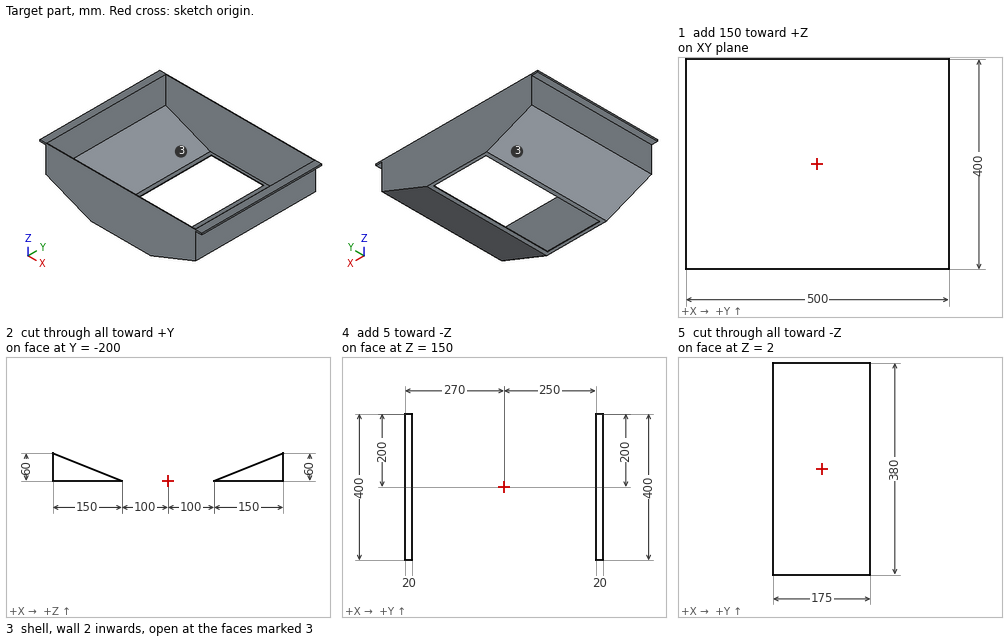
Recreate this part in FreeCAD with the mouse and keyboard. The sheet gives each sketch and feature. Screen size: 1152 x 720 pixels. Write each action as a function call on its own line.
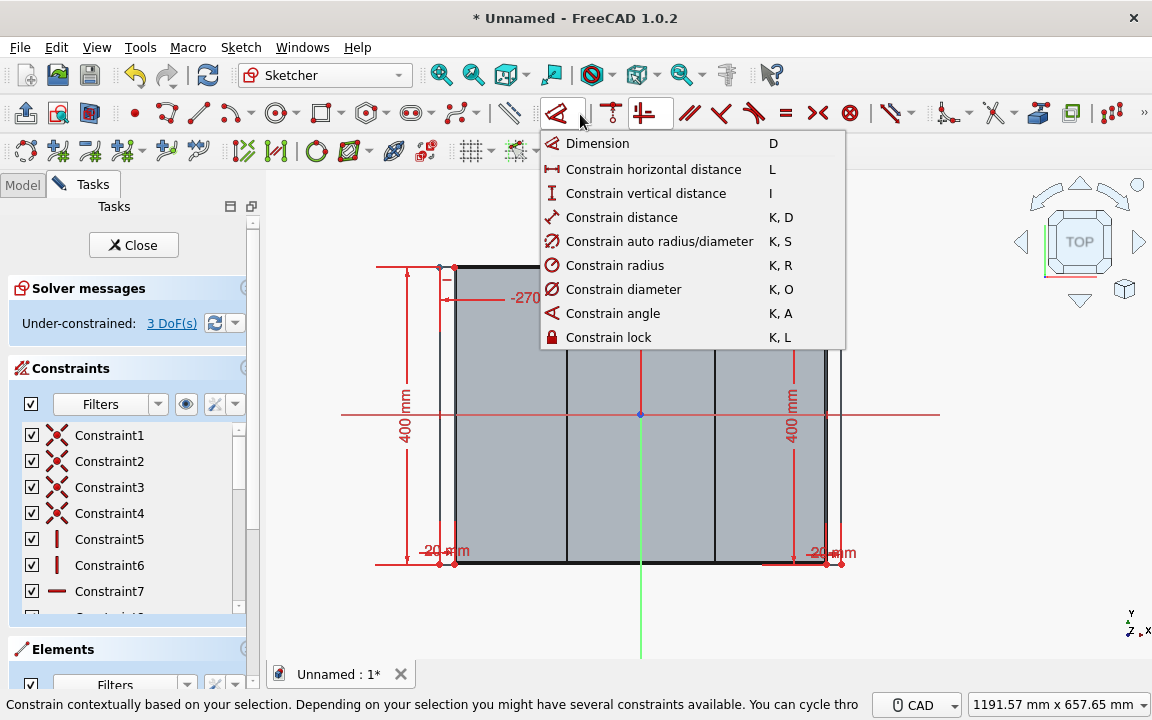
click(693, 193)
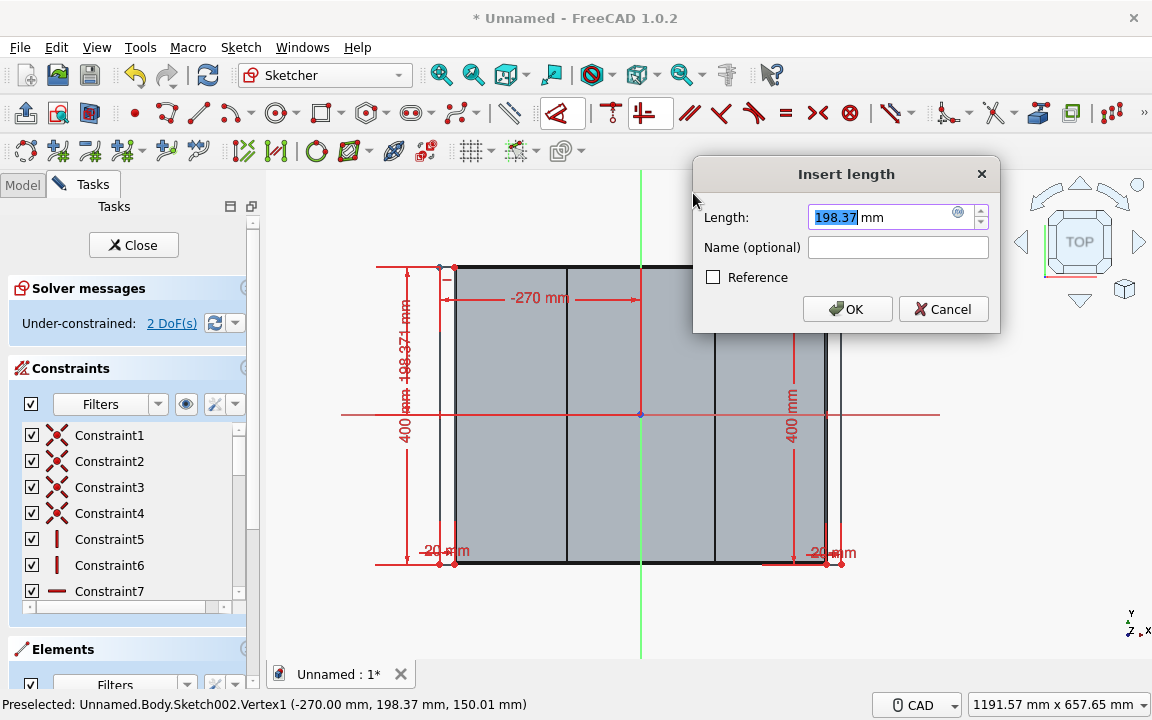
text(200)
key(Return)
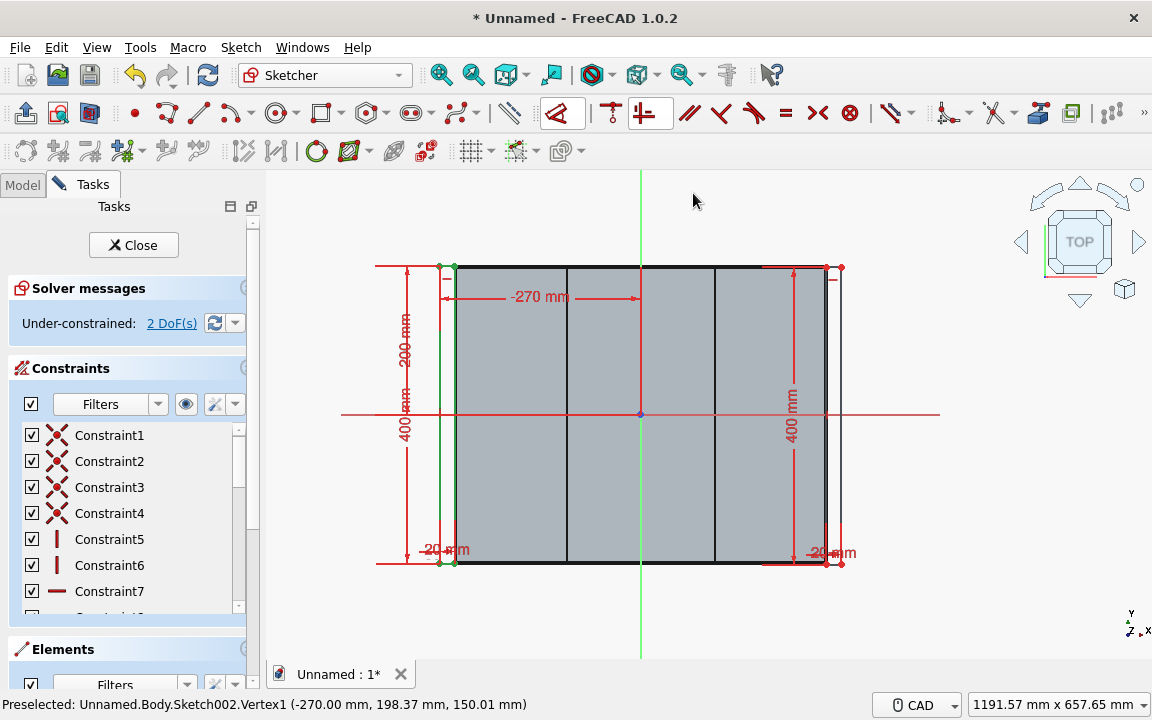
click(826, 267)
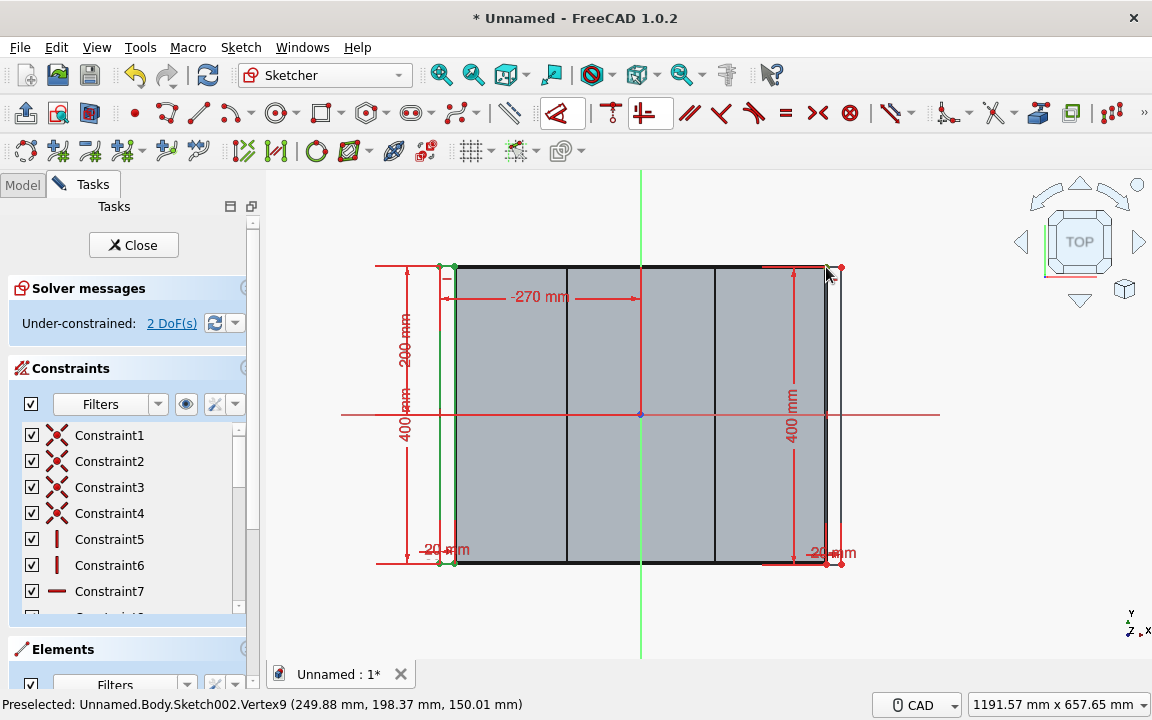
key(l)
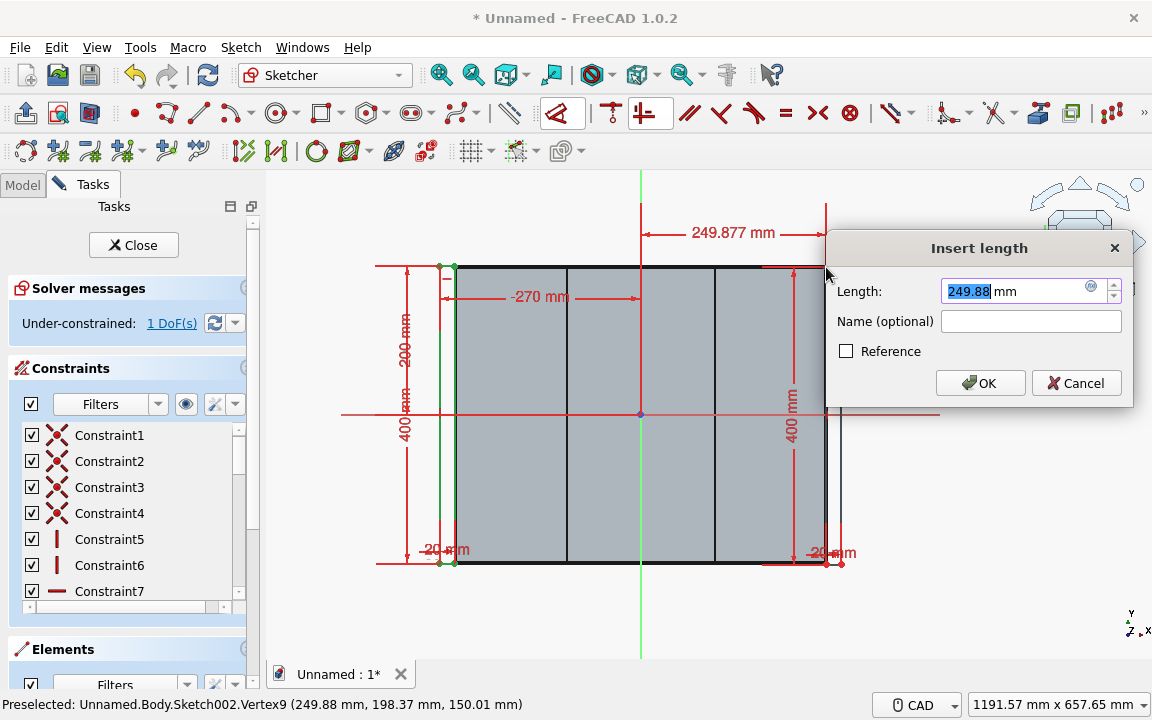
text(250)
key(Return)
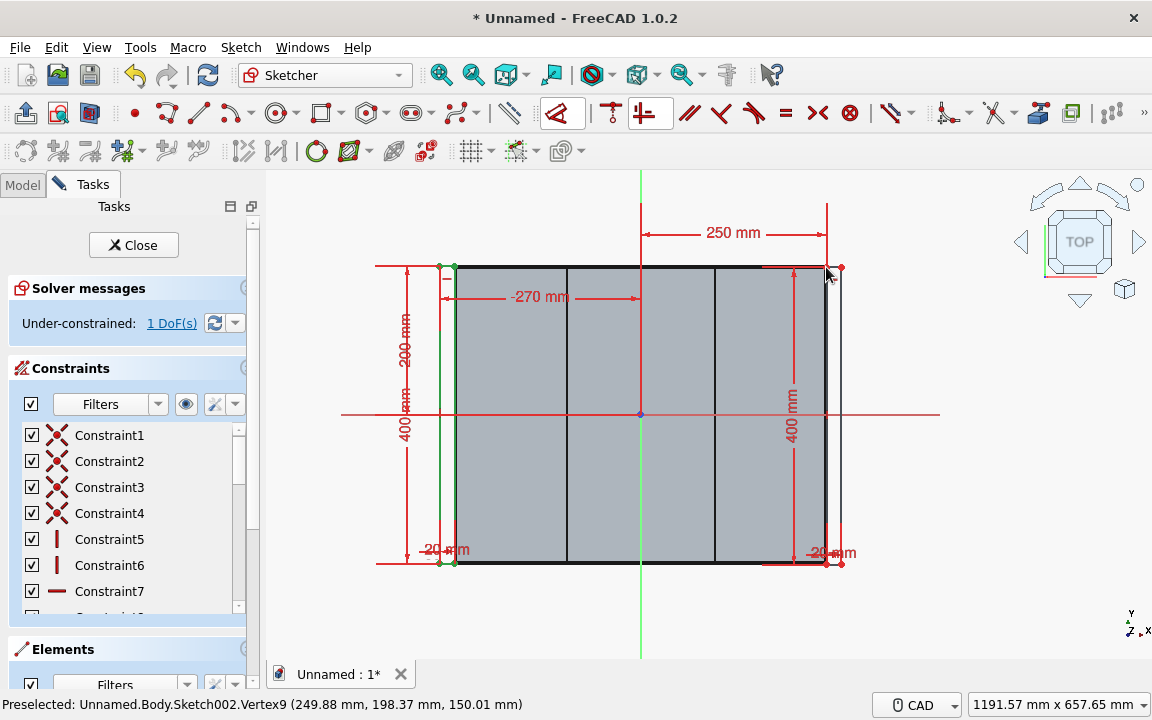
click(827, 267)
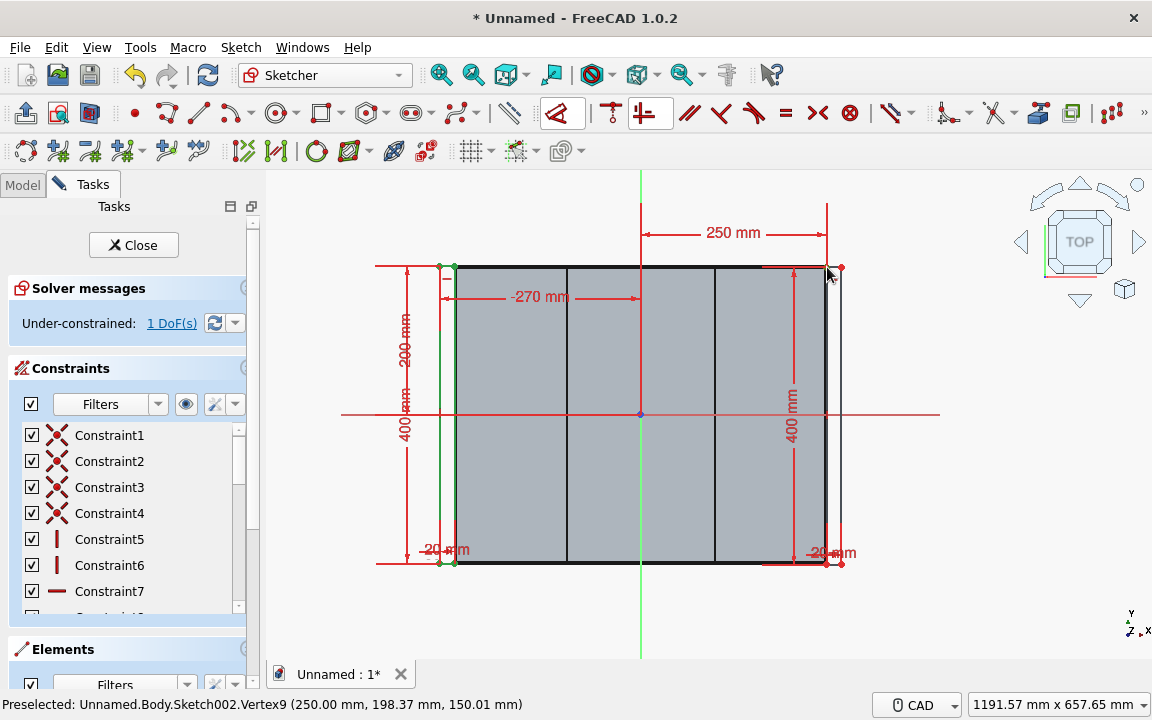
key(i)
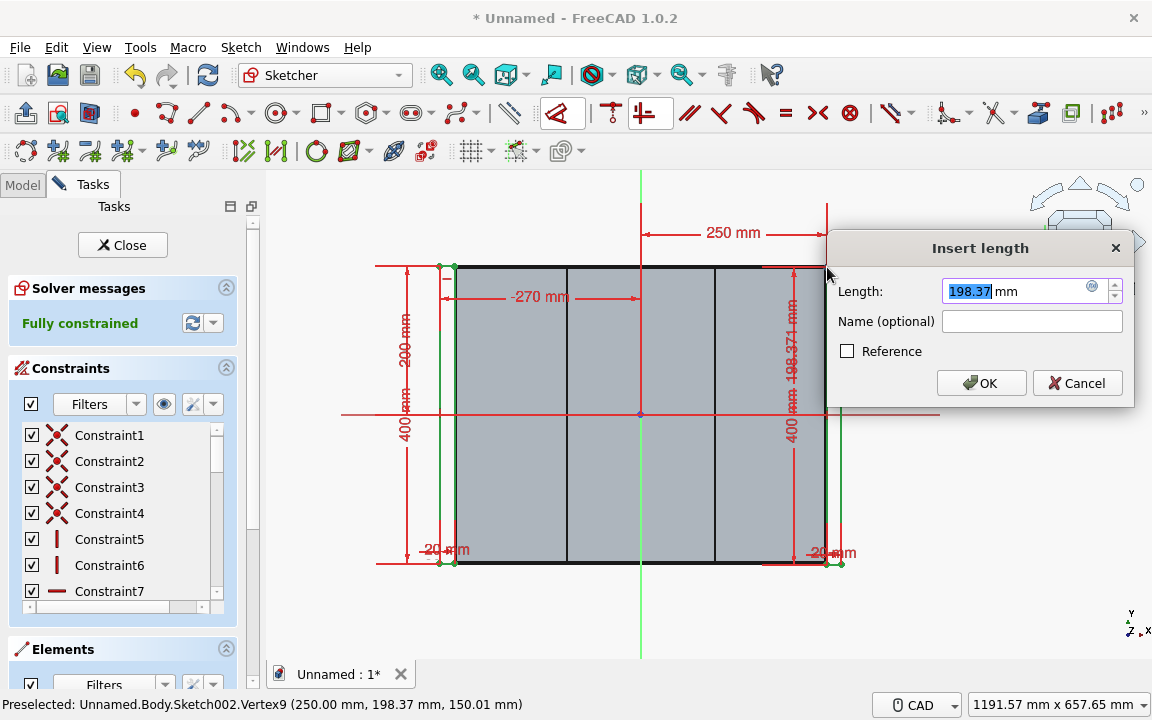
text(200)
key(Return)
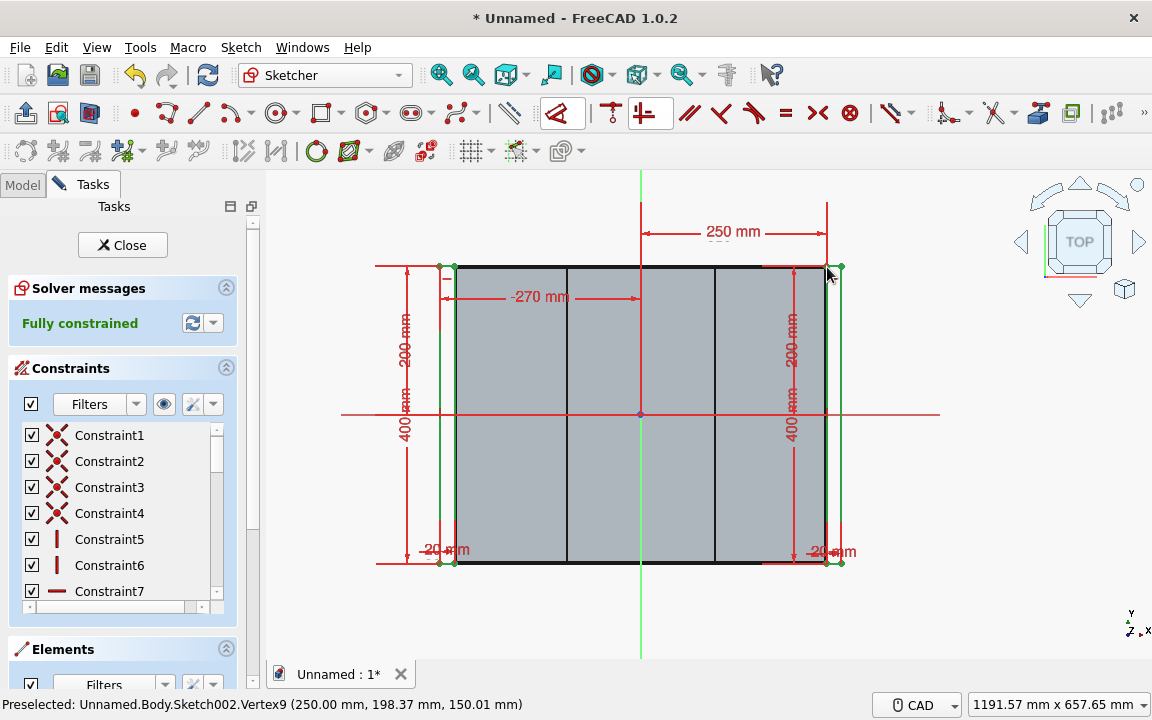
click(123, 245)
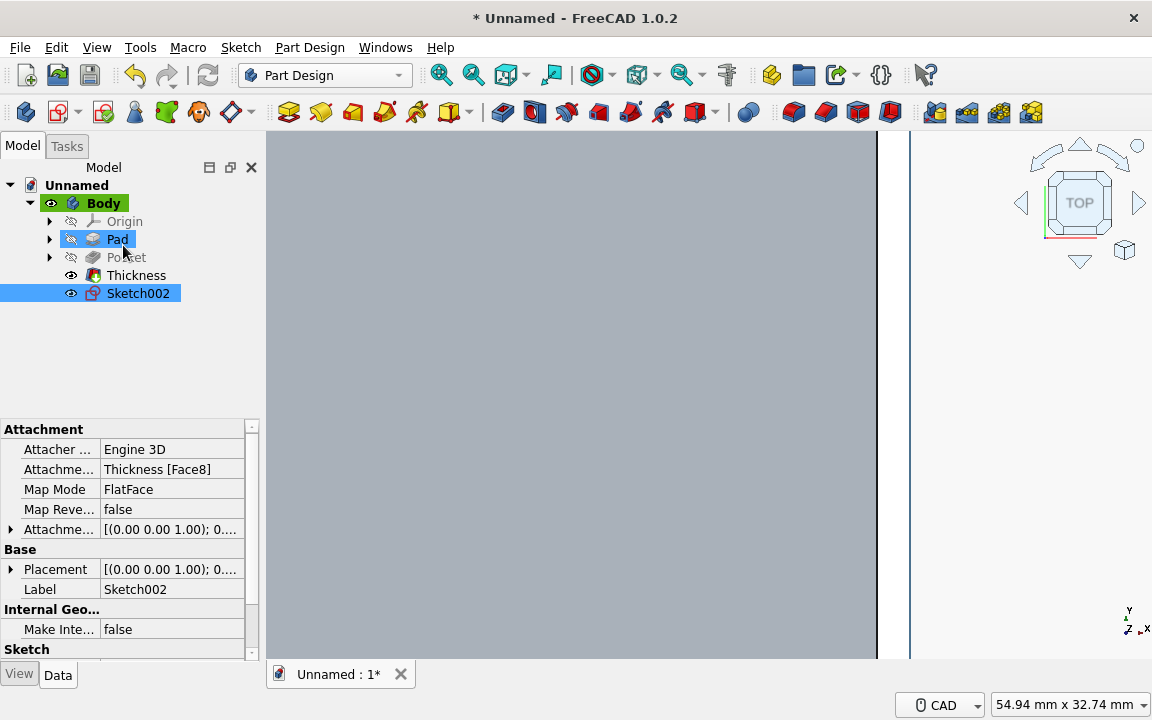
click(290, 112)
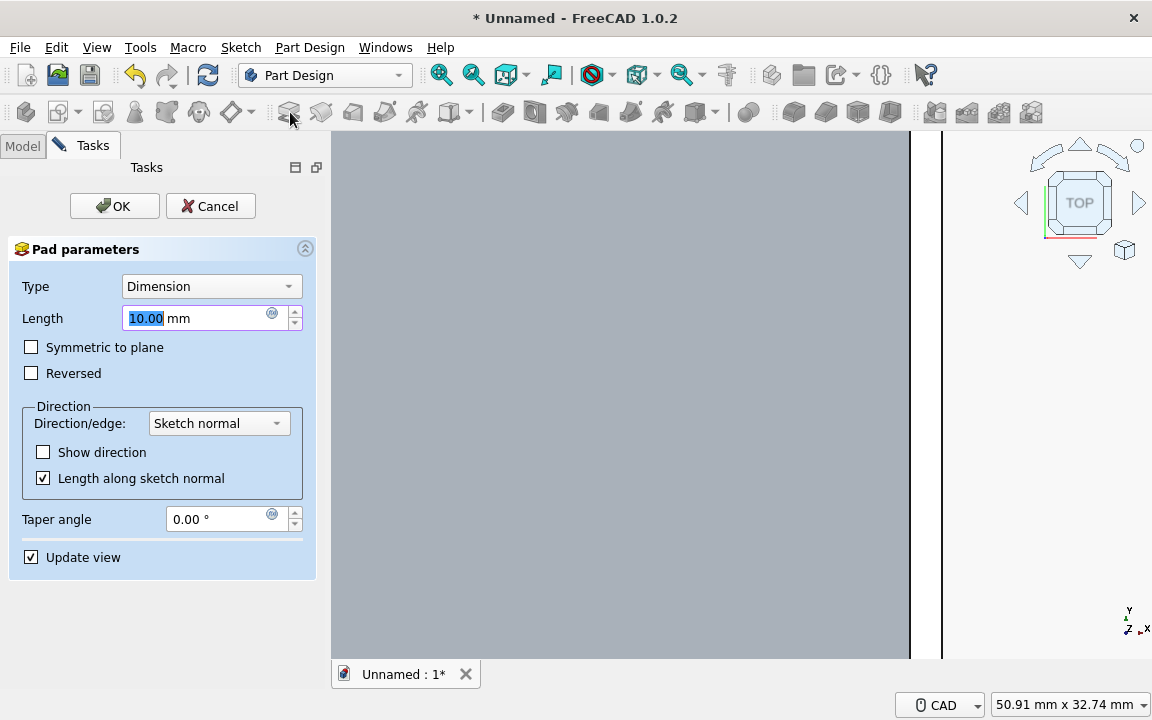
text(5)
key(Tab)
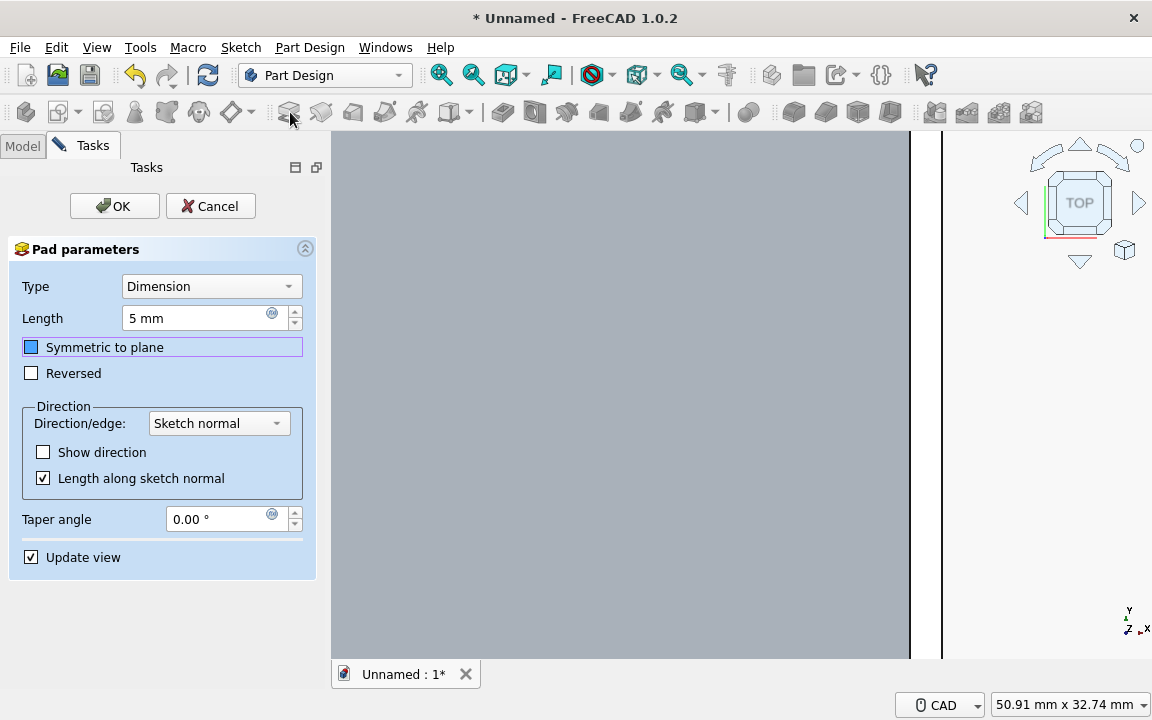
click(30, 373)